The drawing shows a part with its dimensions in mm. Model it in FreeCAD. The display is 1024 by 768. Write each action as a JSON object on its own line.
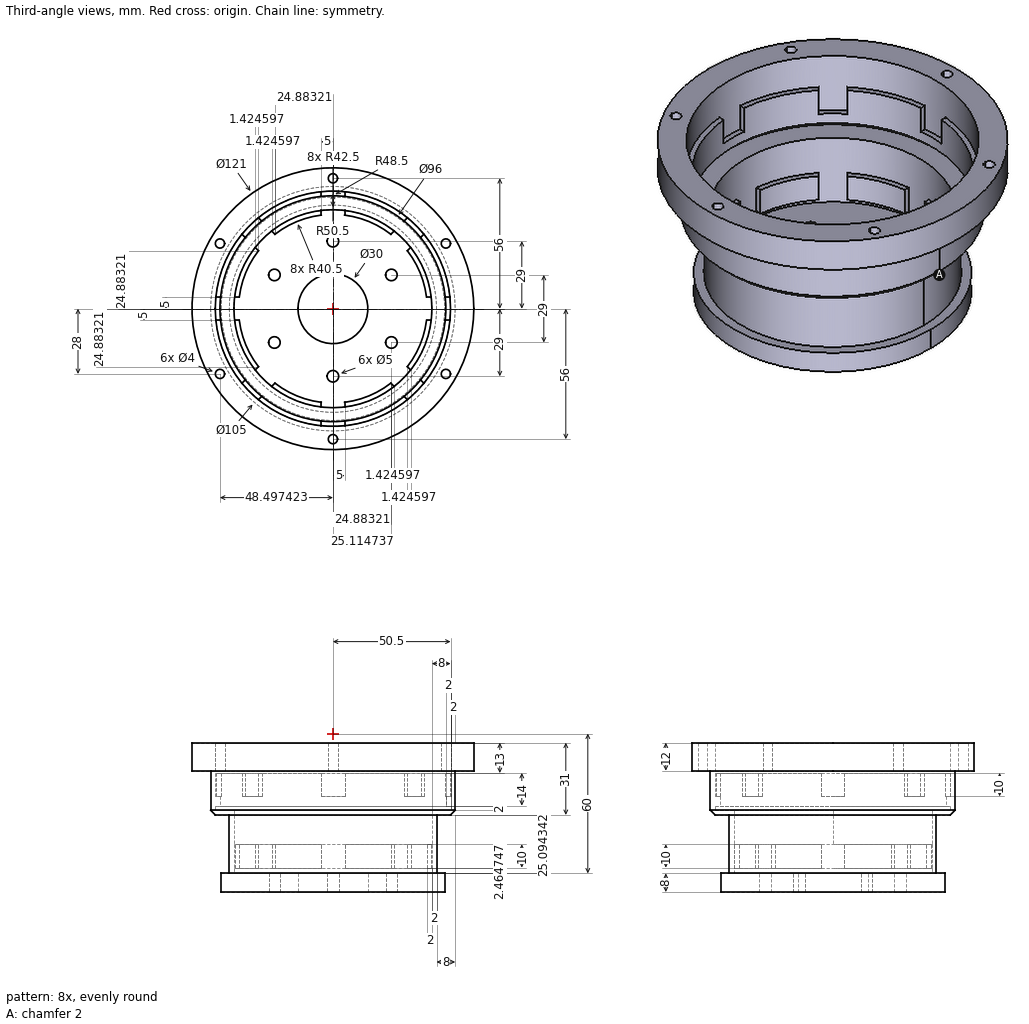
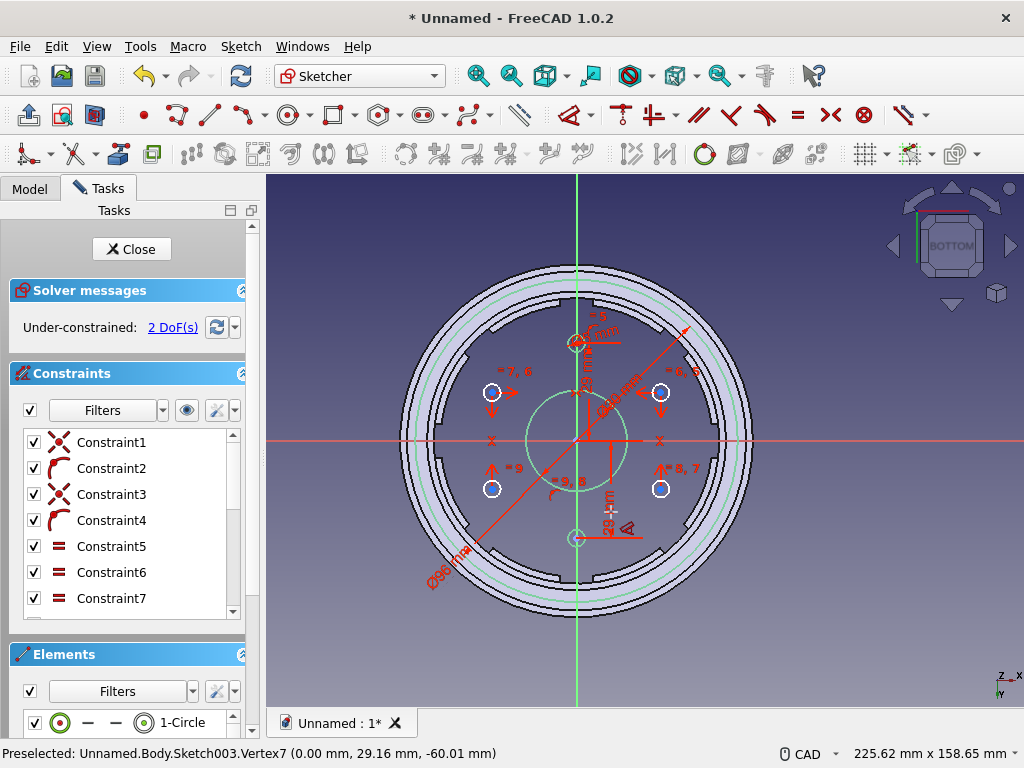
{"action": "left_click", "coordinate": [661, 393]}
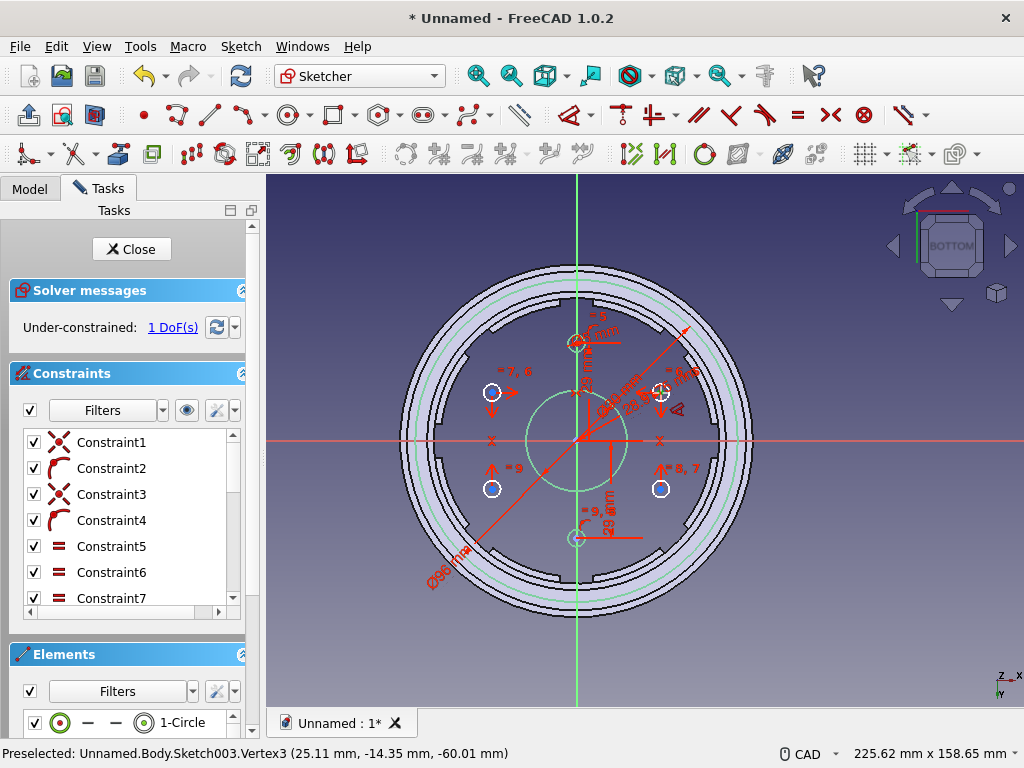
{"action": "left_click", "coordinate": [661, 489]}
{"action": "left_click", "coordinate": [695, 419]}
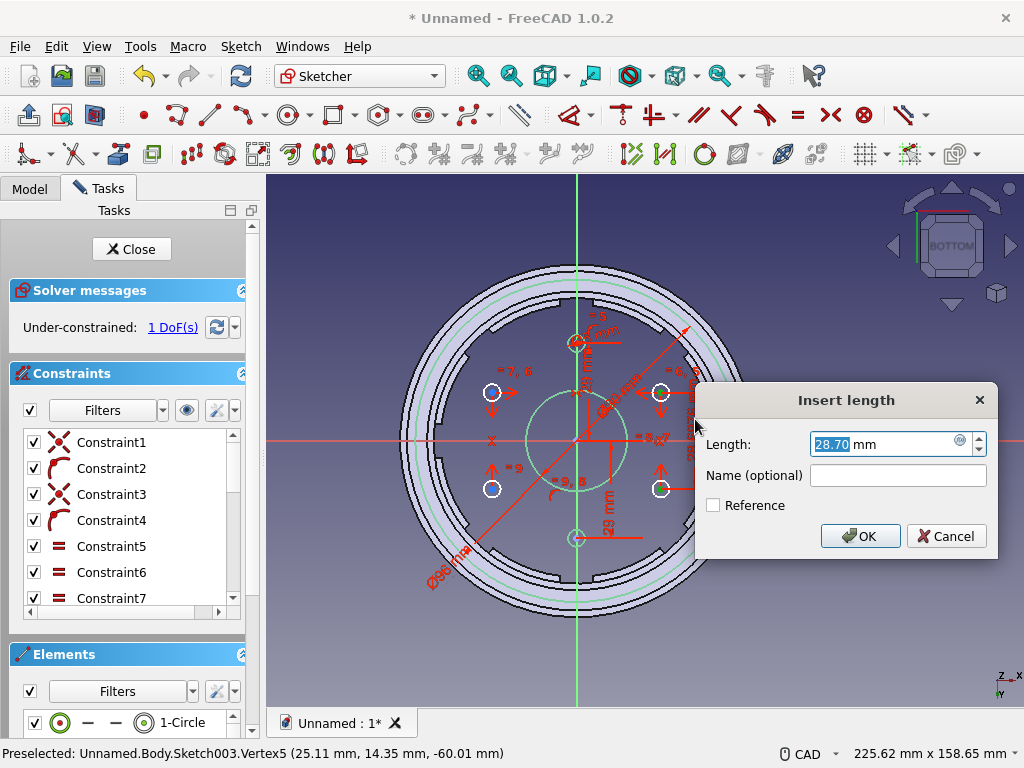
{"action": "type", "text": "29"}
{"action": "key", "text": "Return"}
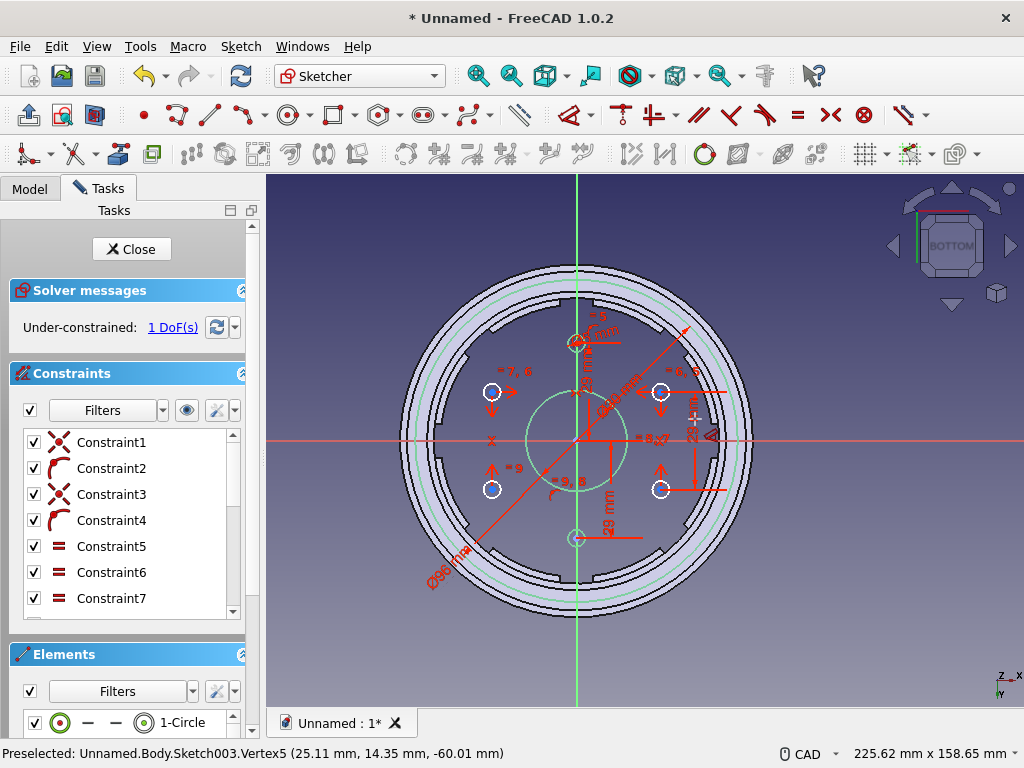
{"action": "left_click", "coordinate": [661, 392]}
{"action": "left_click", "coordinate": [638, 475]}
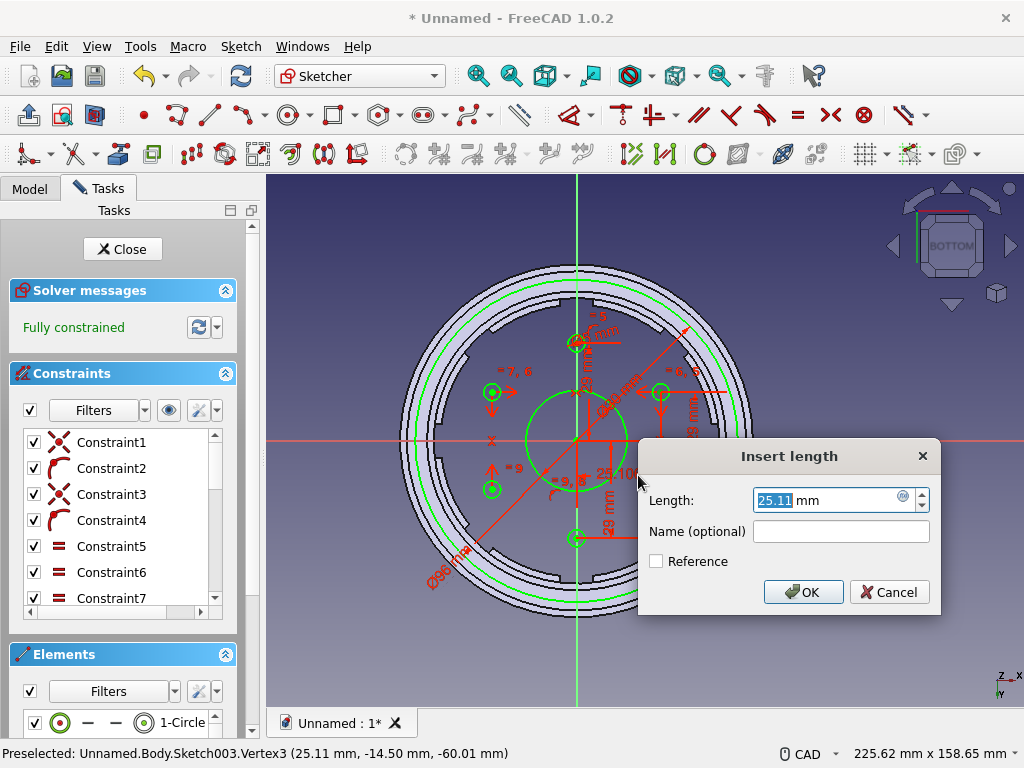
{"action": "type", "text": "25.114737"}
{"action": "key", "text": "Return"}
{"action": "key", "text": "Escape"}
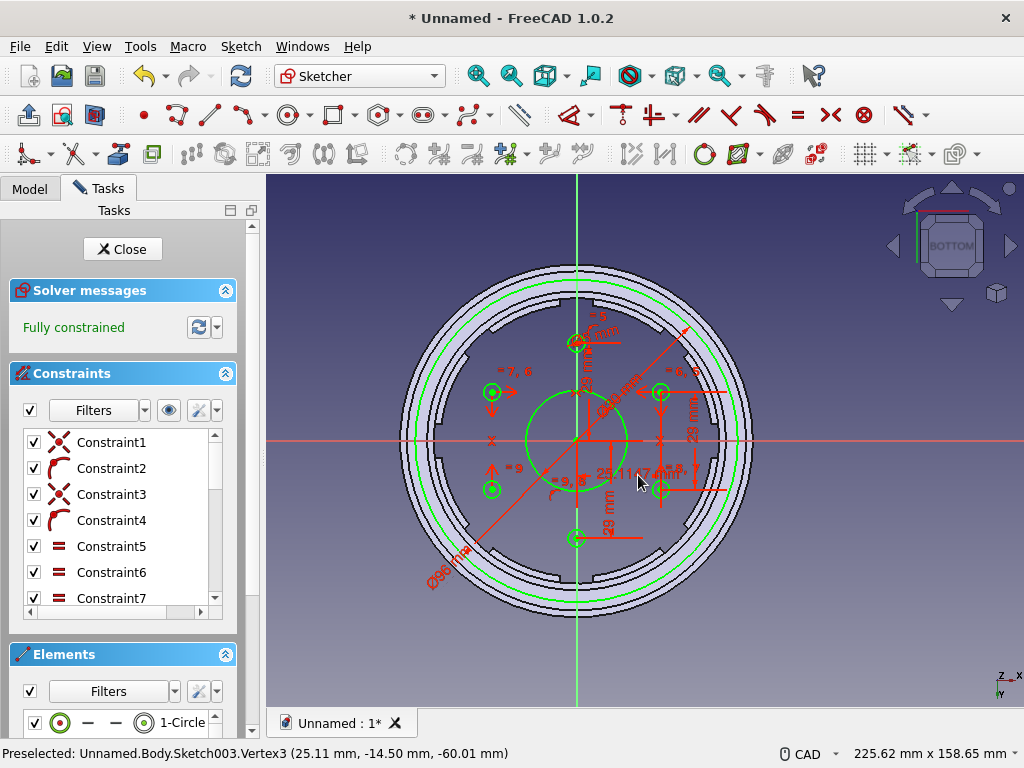
{"action": "left_click", "coordinate": [123, 249]}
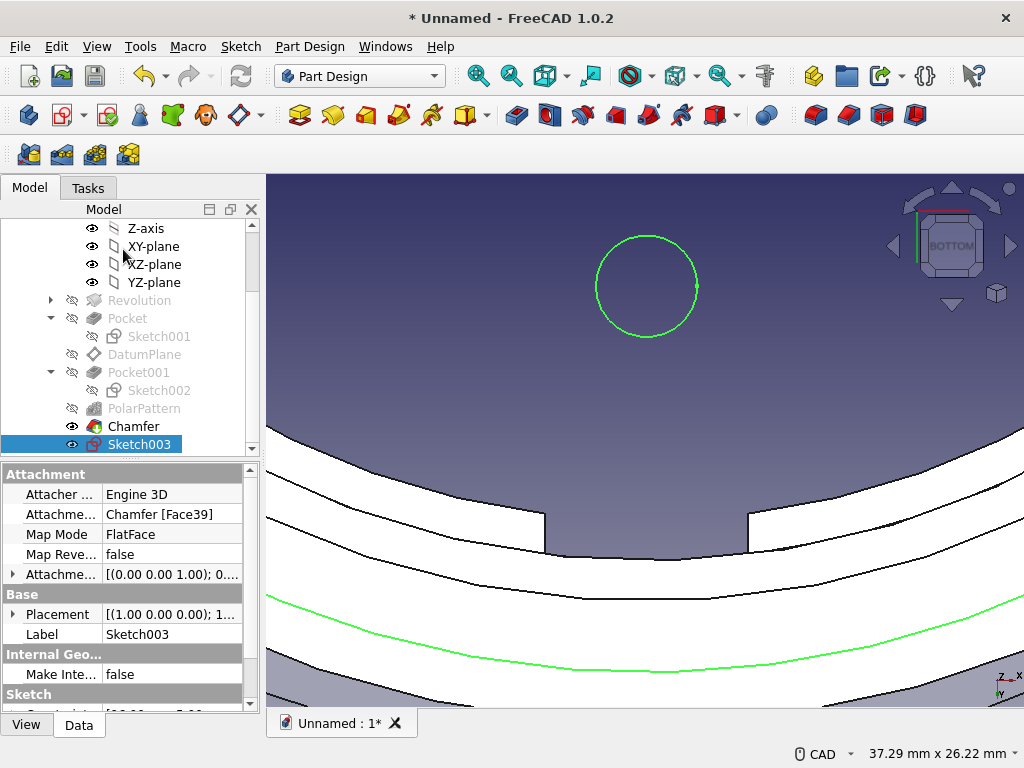
{"action": "left_click", "coordinate": [300, 116]}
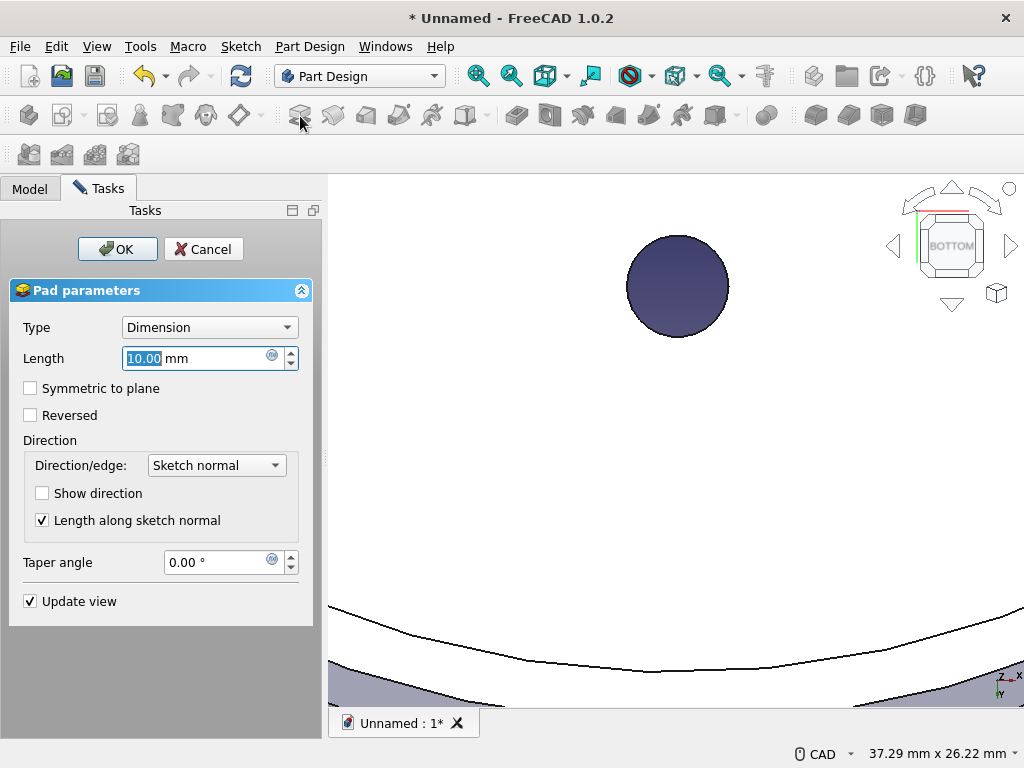
{"action": "type", "text": "8"}
{"action": "key", "text": "Tab"}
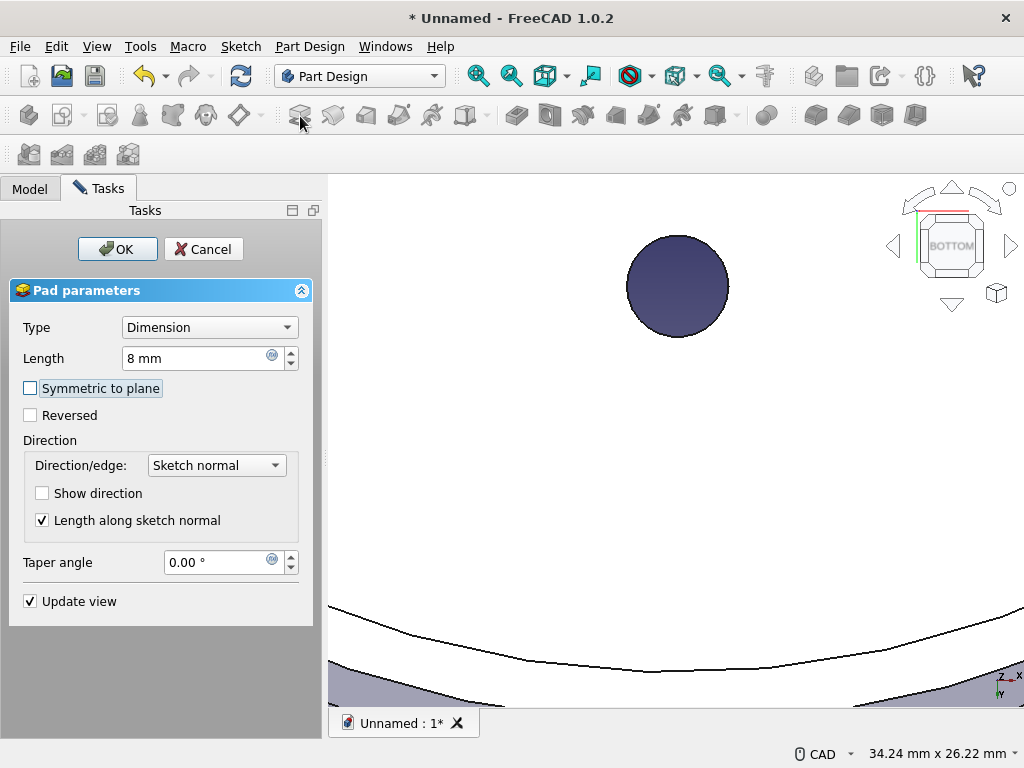
{"action": "left_click", "coordinate": [118, 249]}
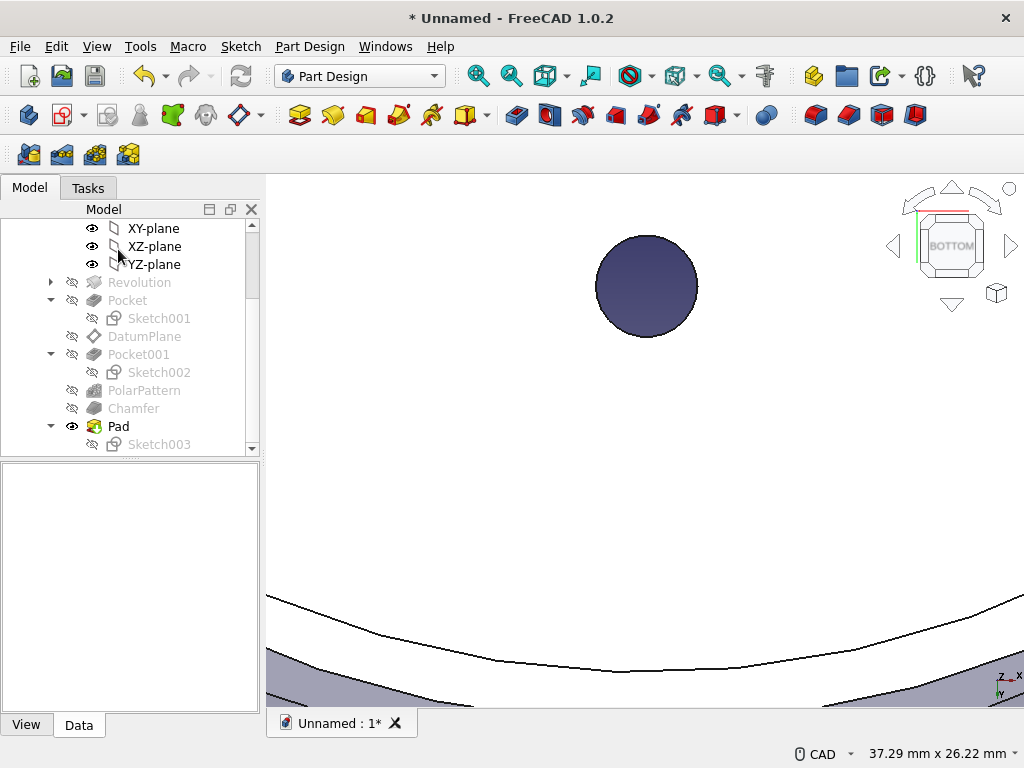
{"action": "left_click", "coordinate": [479, 76]}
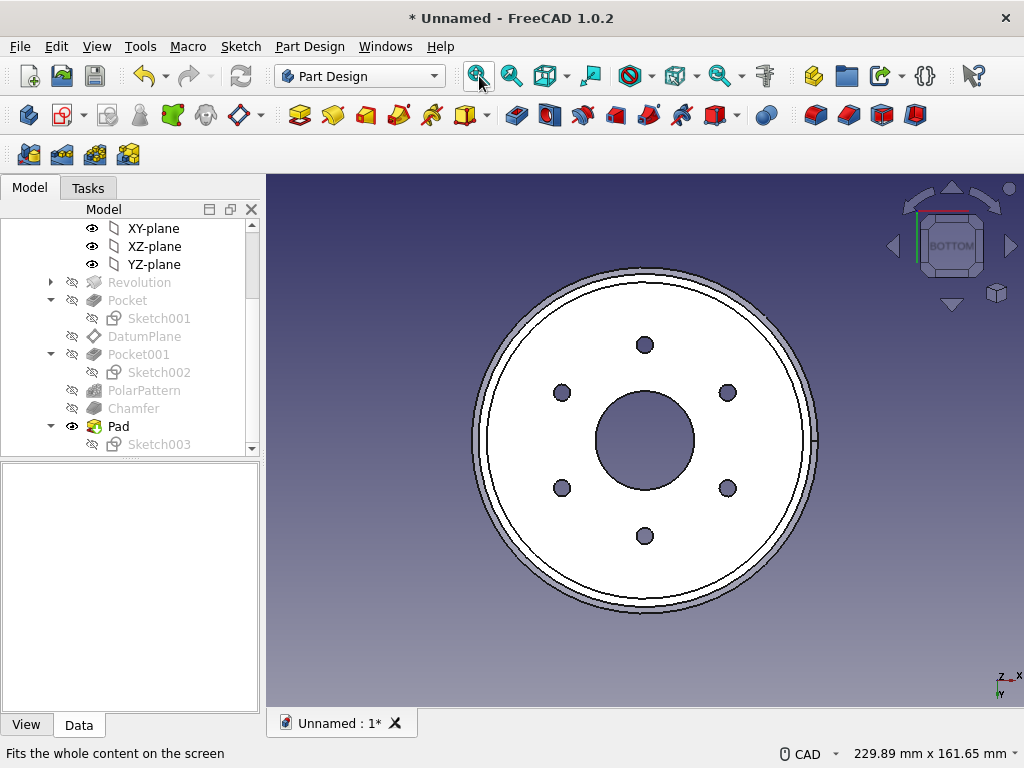
{"action": "key", "text": "0"}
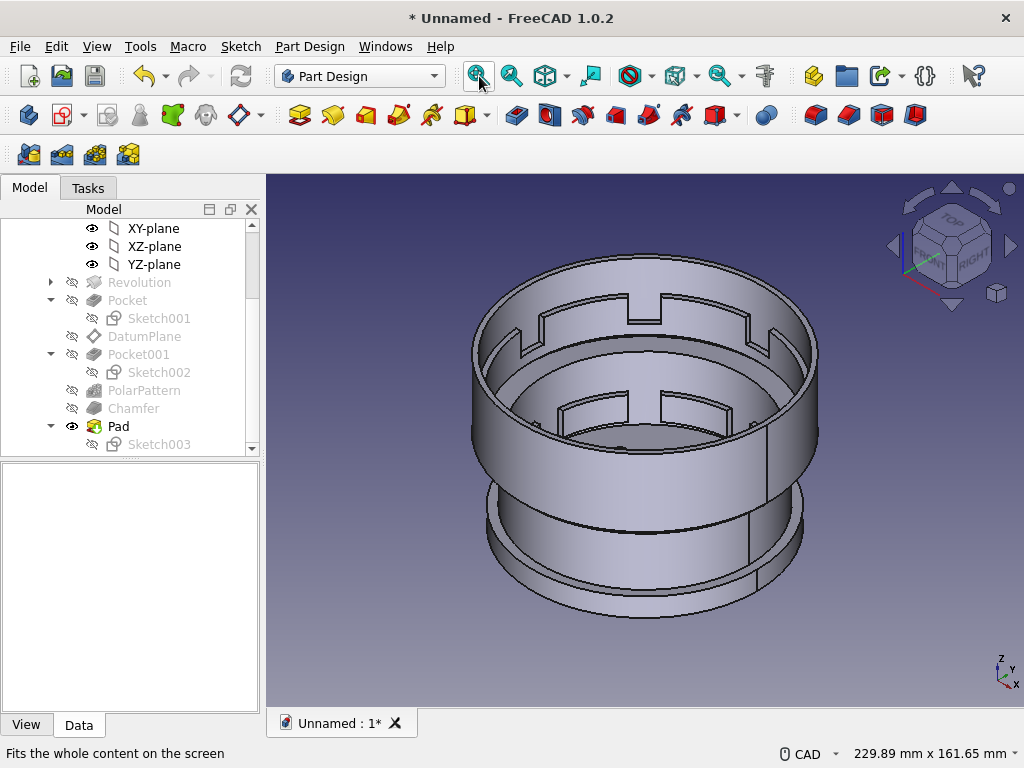
{"action": "scroll", "coordinate": [816, 355], "scroll_direction": "up", "scroll_amount": 9}